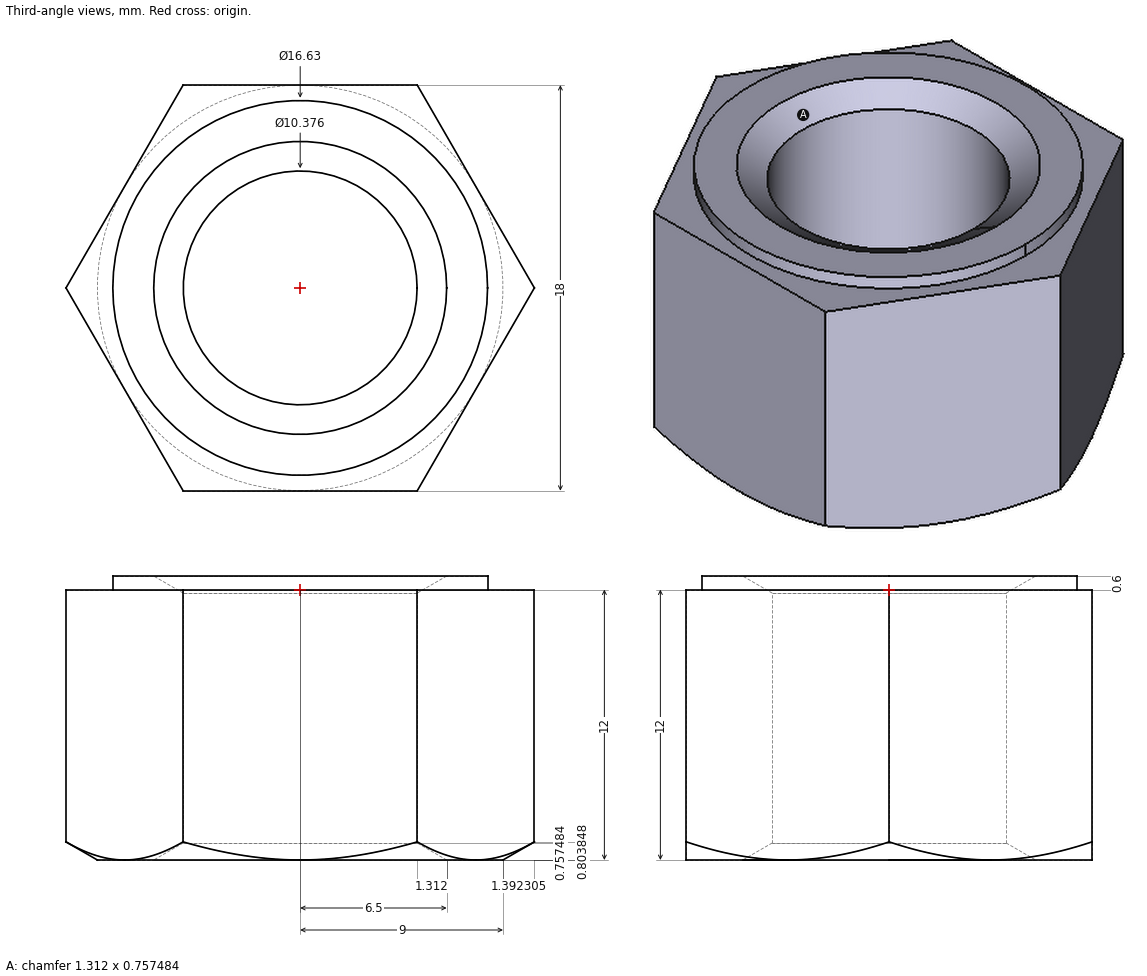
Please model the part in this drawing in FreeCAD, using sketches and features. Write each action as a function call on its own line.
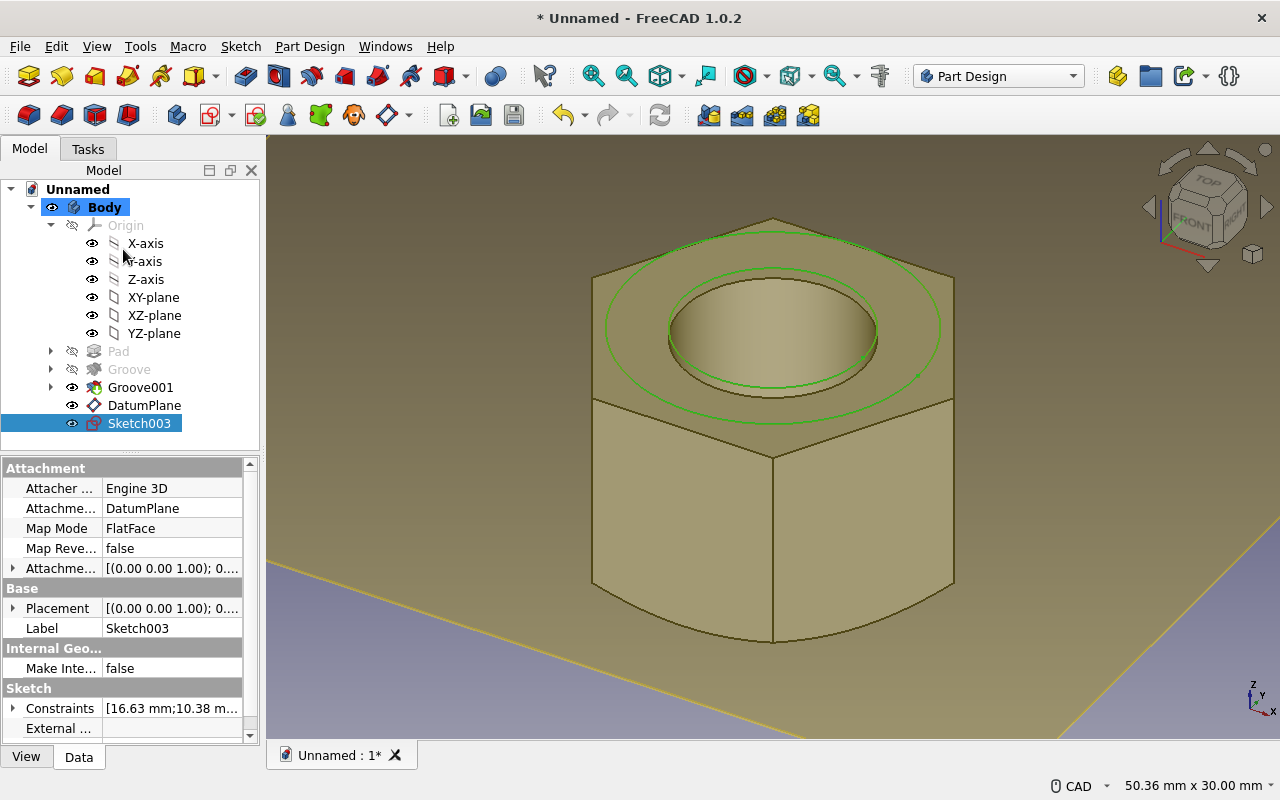
click(29, 76)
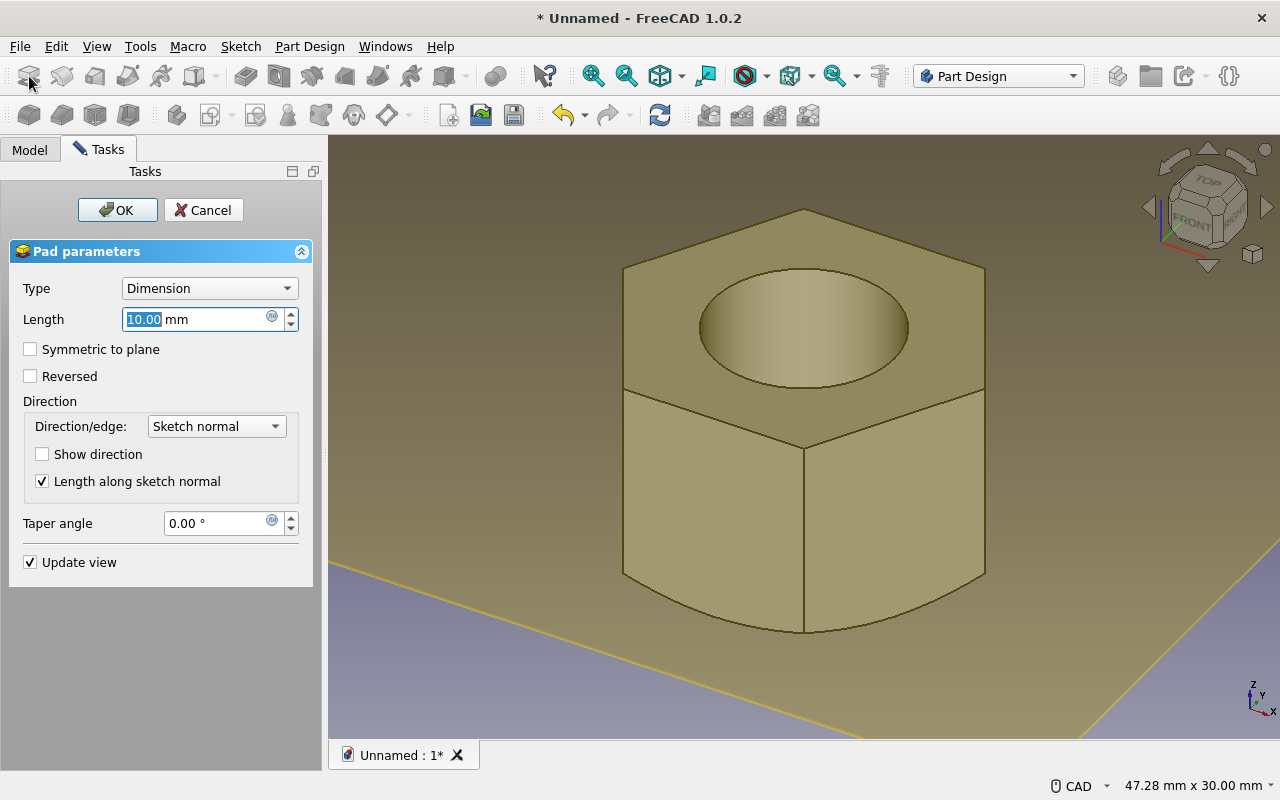
text(0.6)
key(Tab)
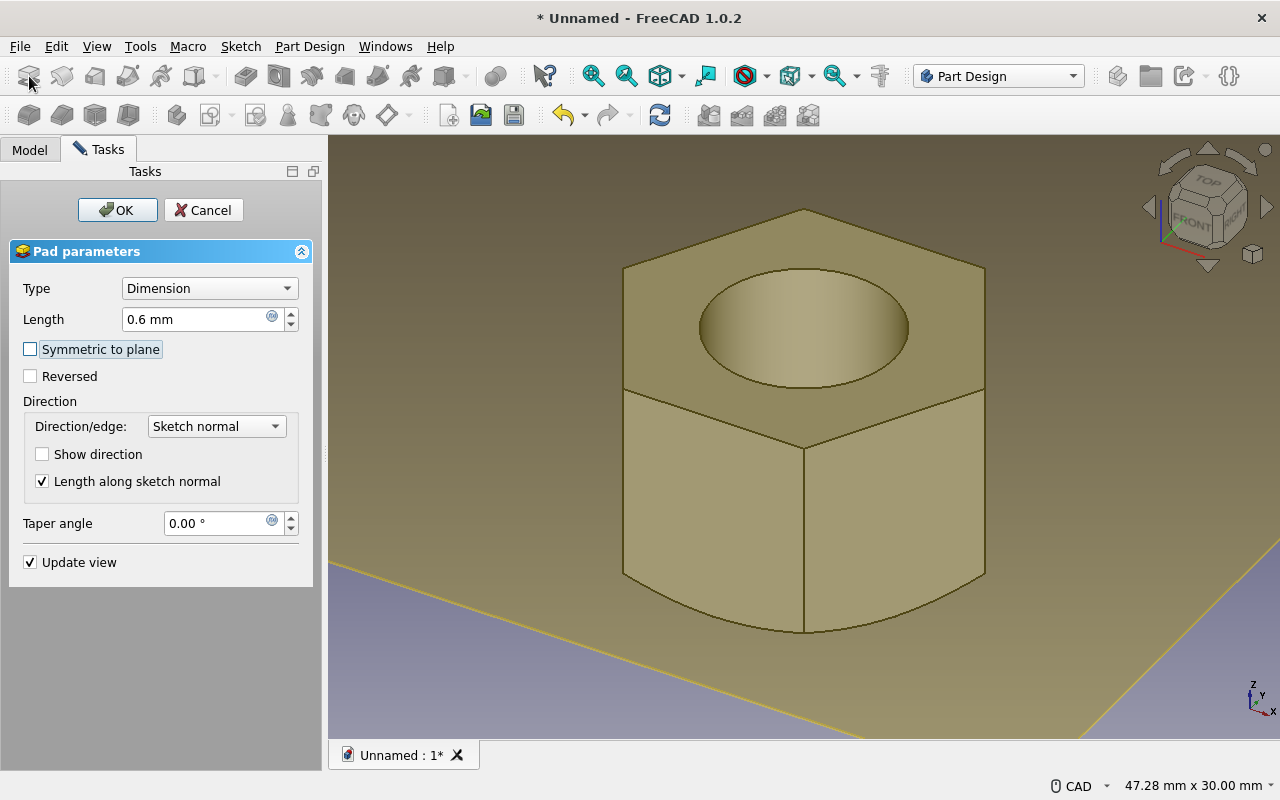
click(31, 376)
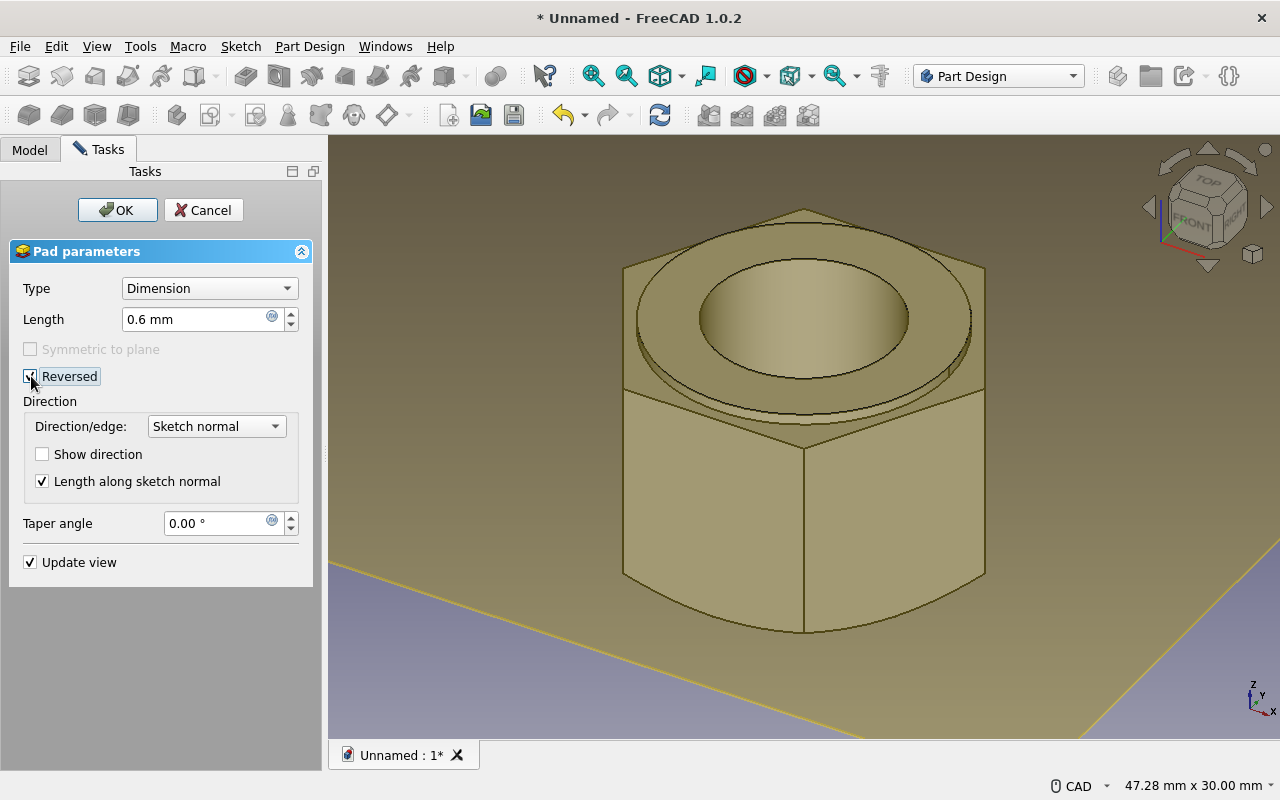
click(118, 210)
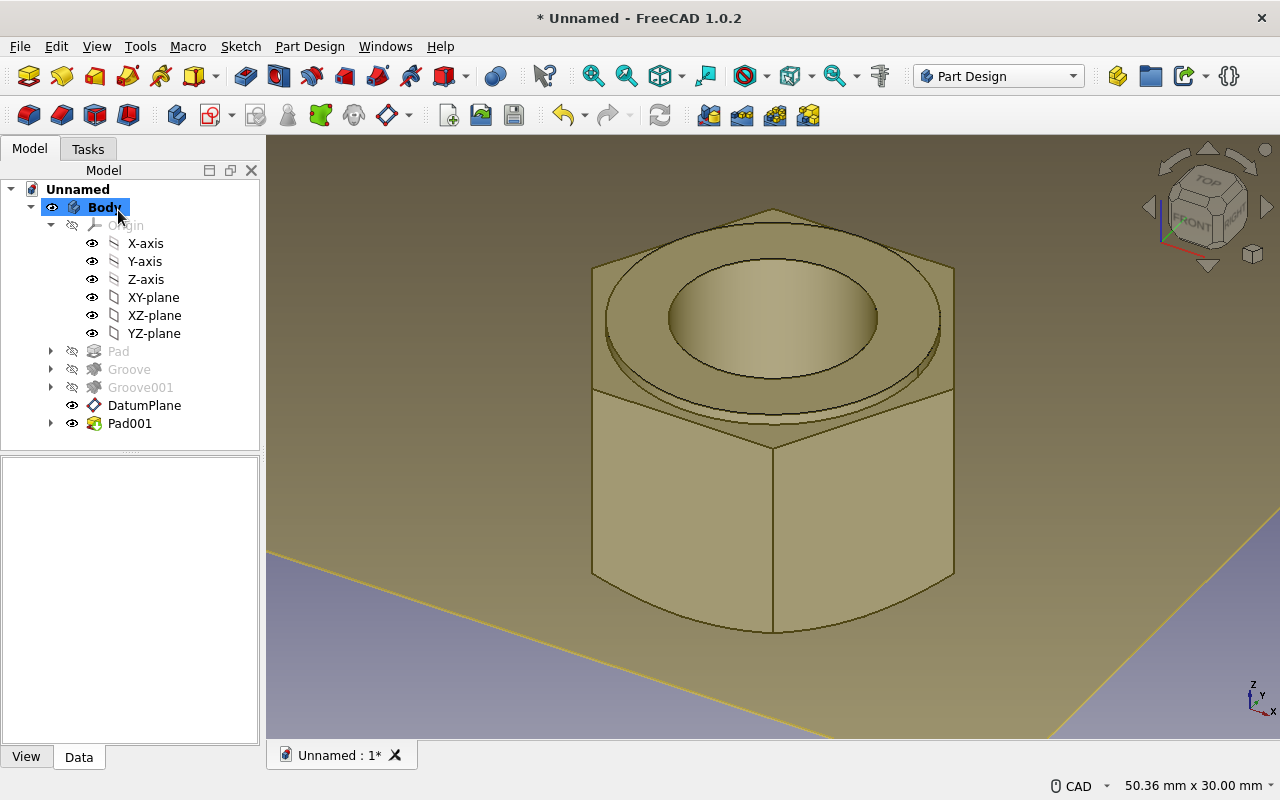
click(117, 405)
key(space)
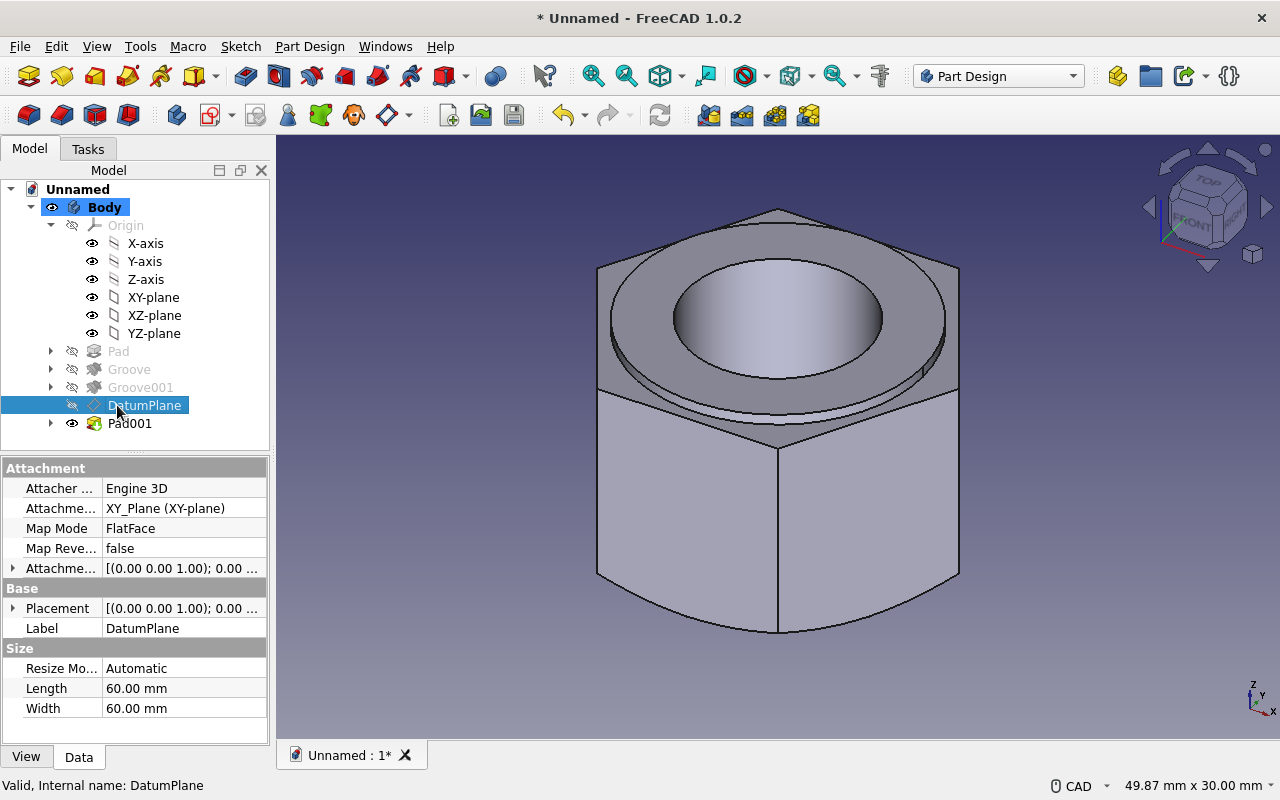
click(688, 288)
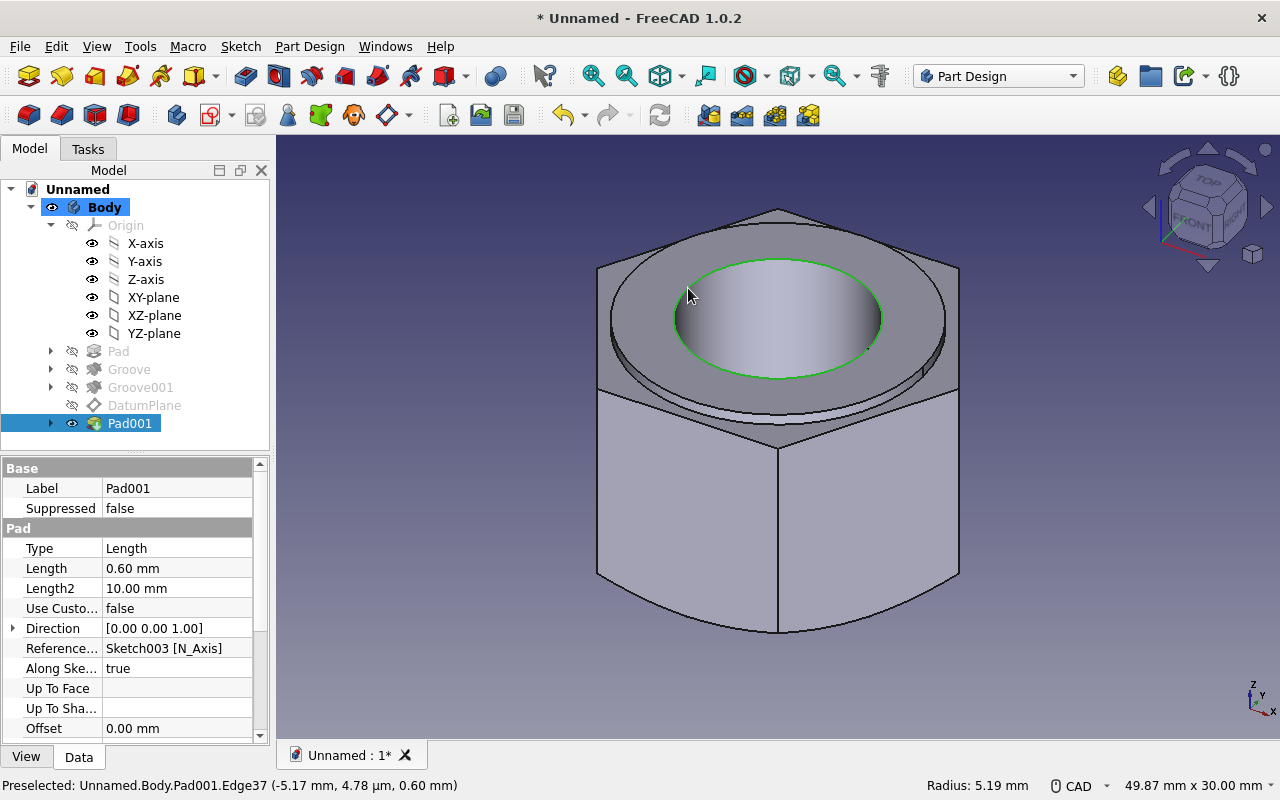
click(62, 116)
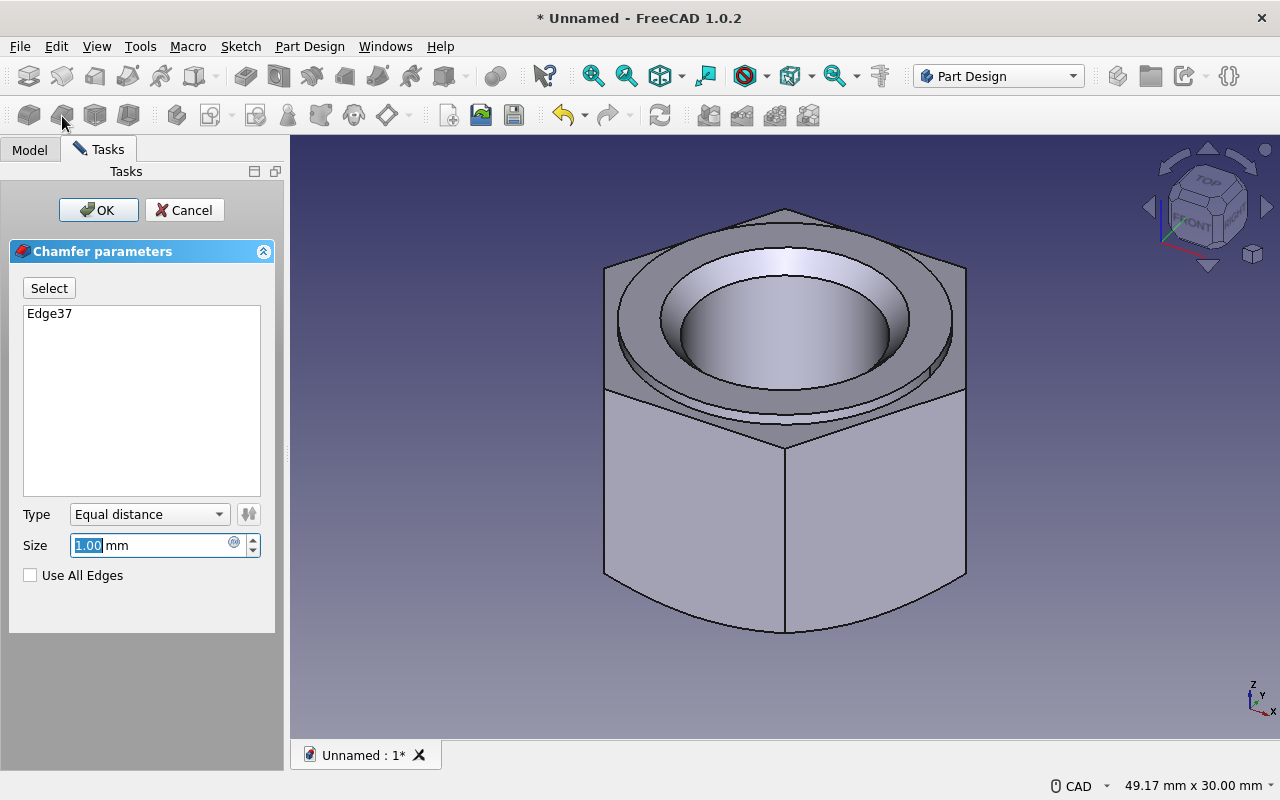
text(1.312)
key(Tab)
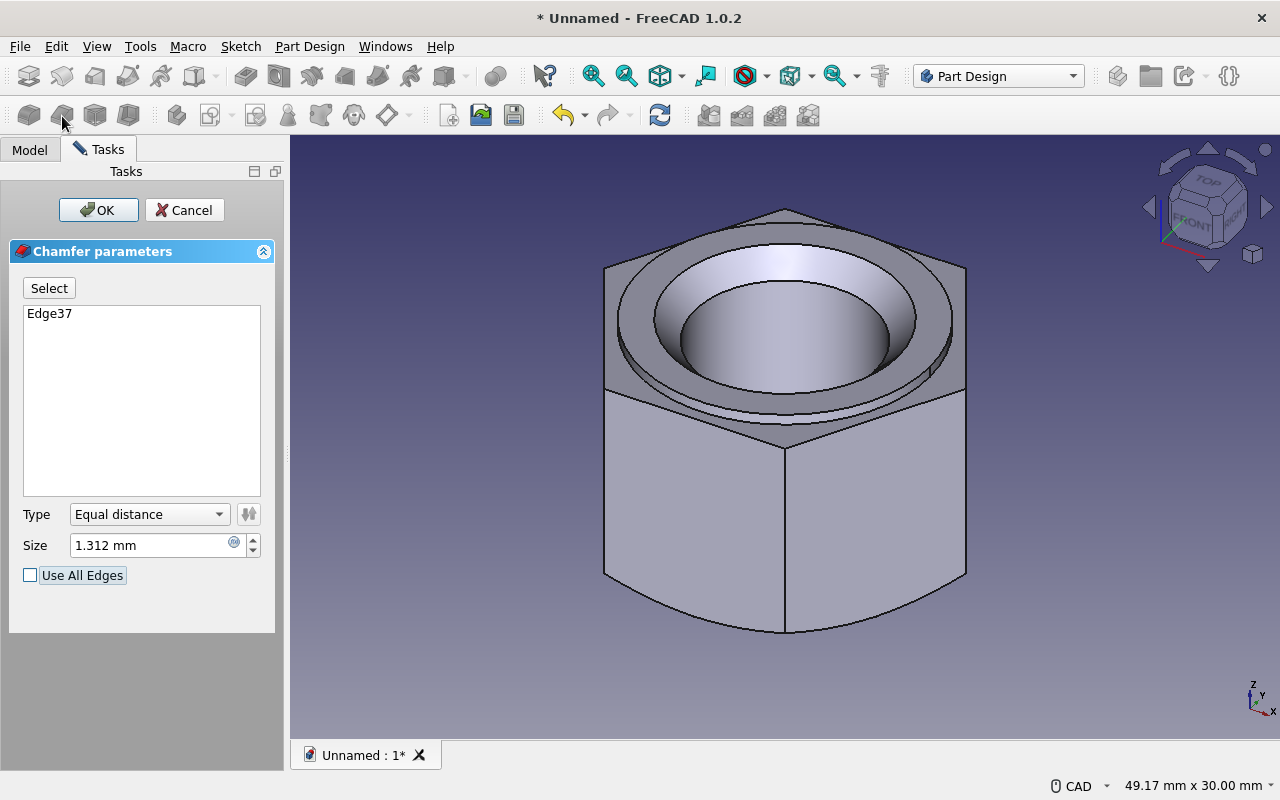
click(150, 514)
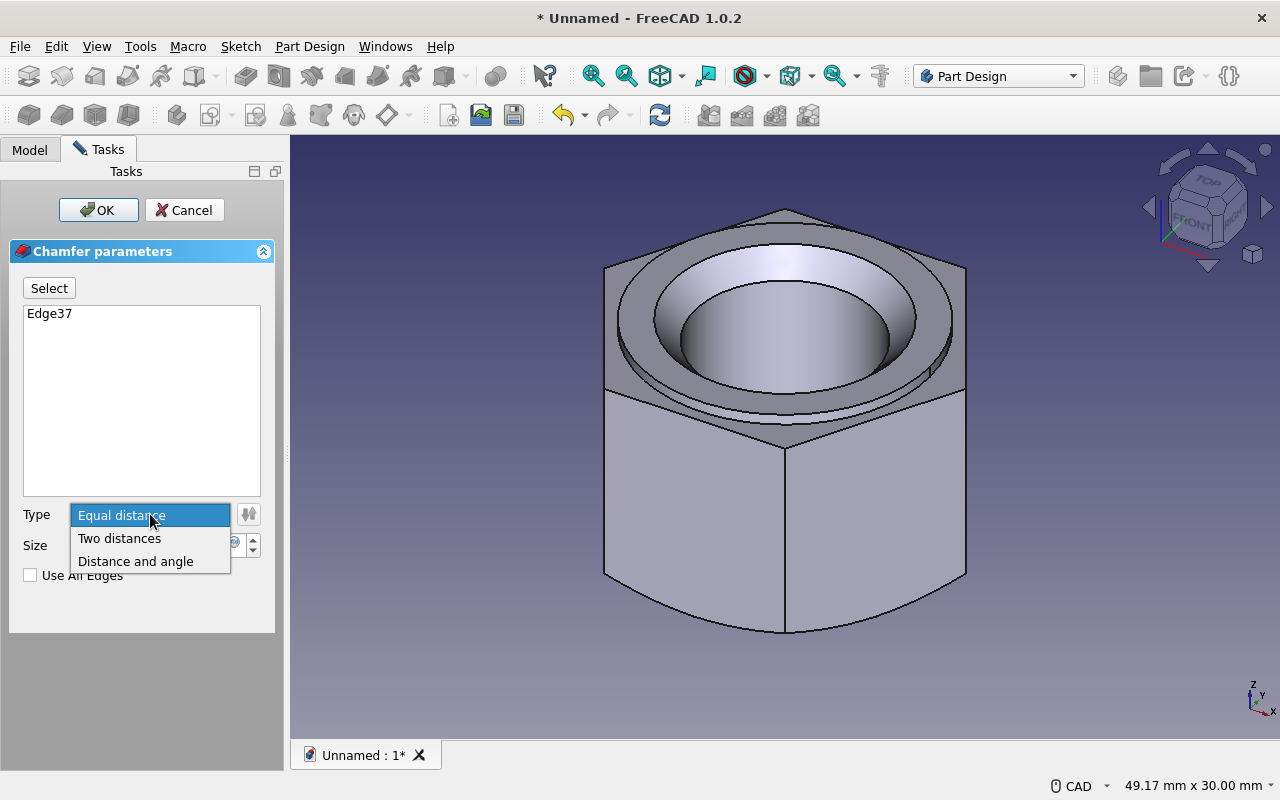
click(148, 538)